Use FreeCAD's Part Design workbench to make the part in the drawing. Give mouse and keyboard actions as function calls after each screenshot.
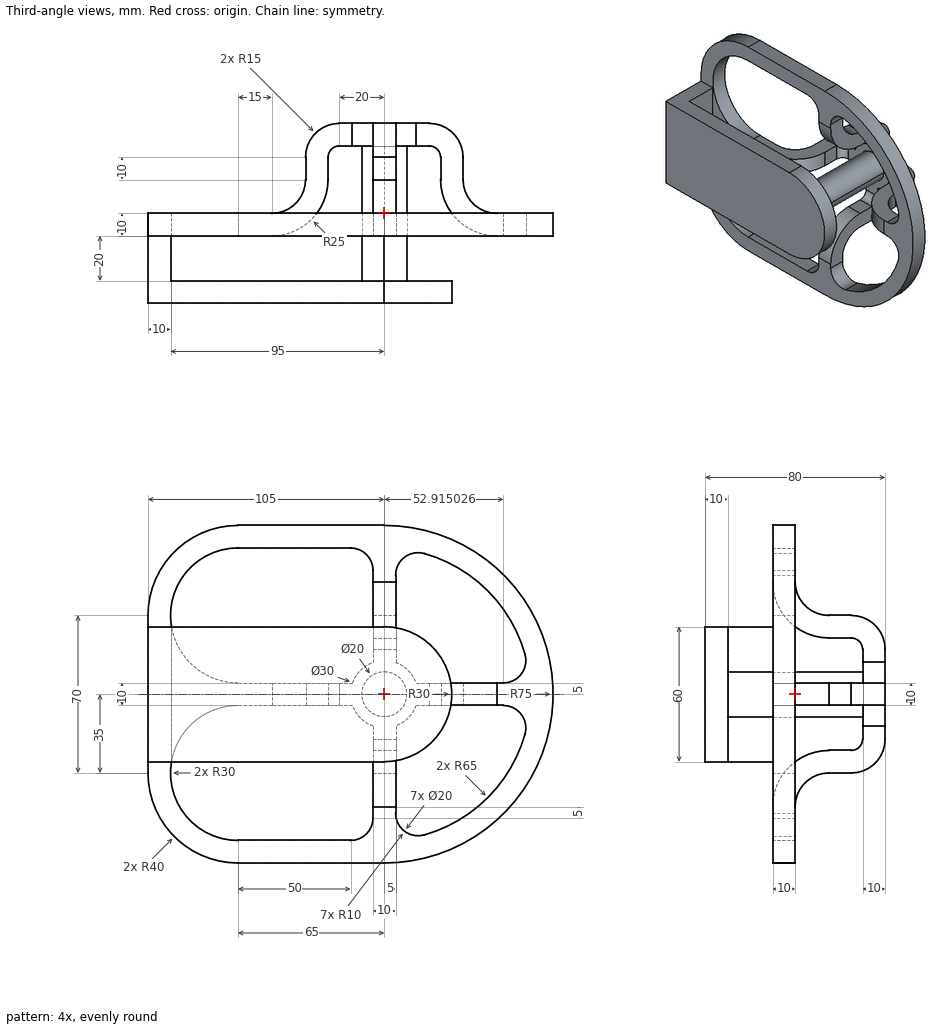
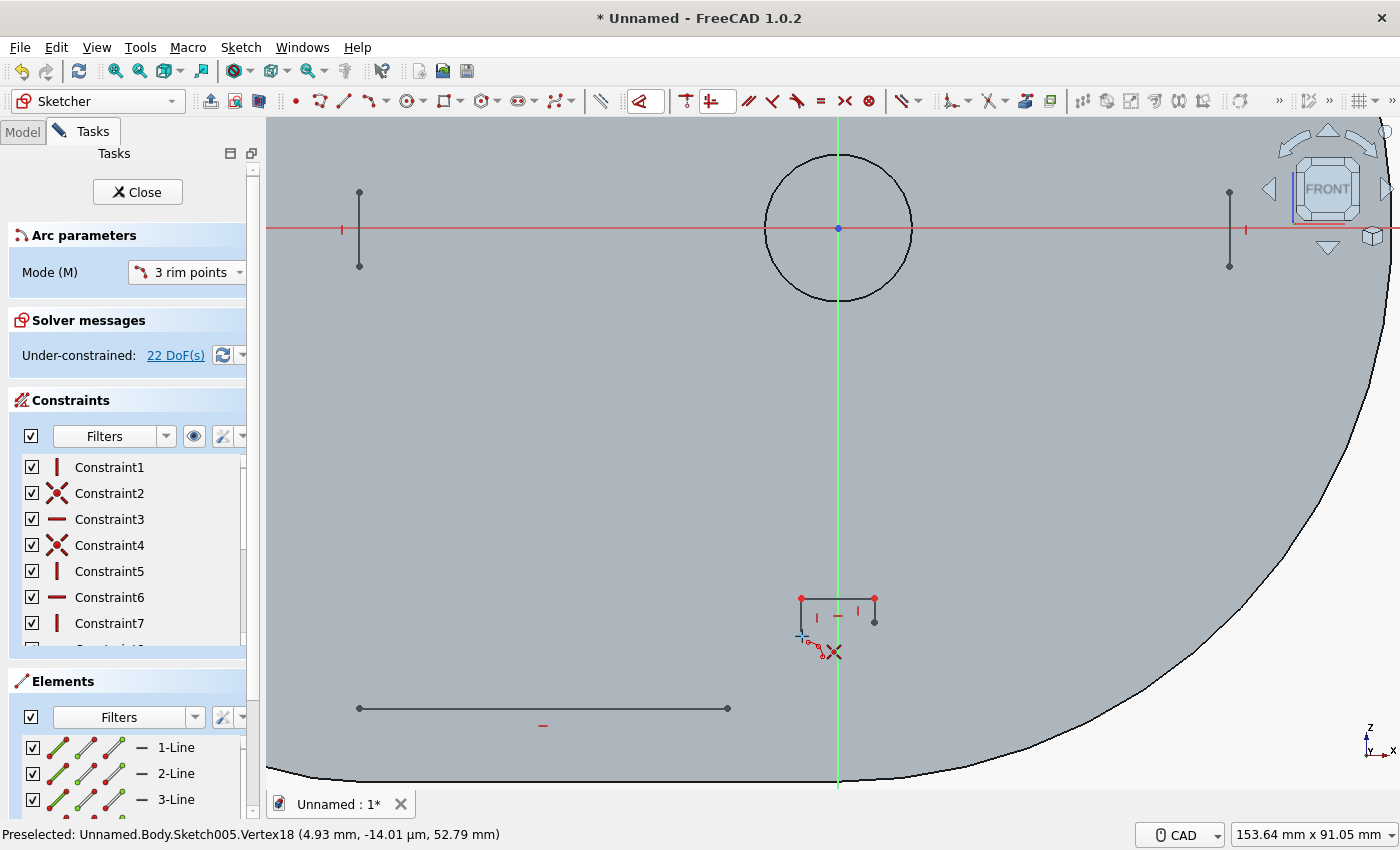
click(801, 635)
click(728, 709)
click(780, 686)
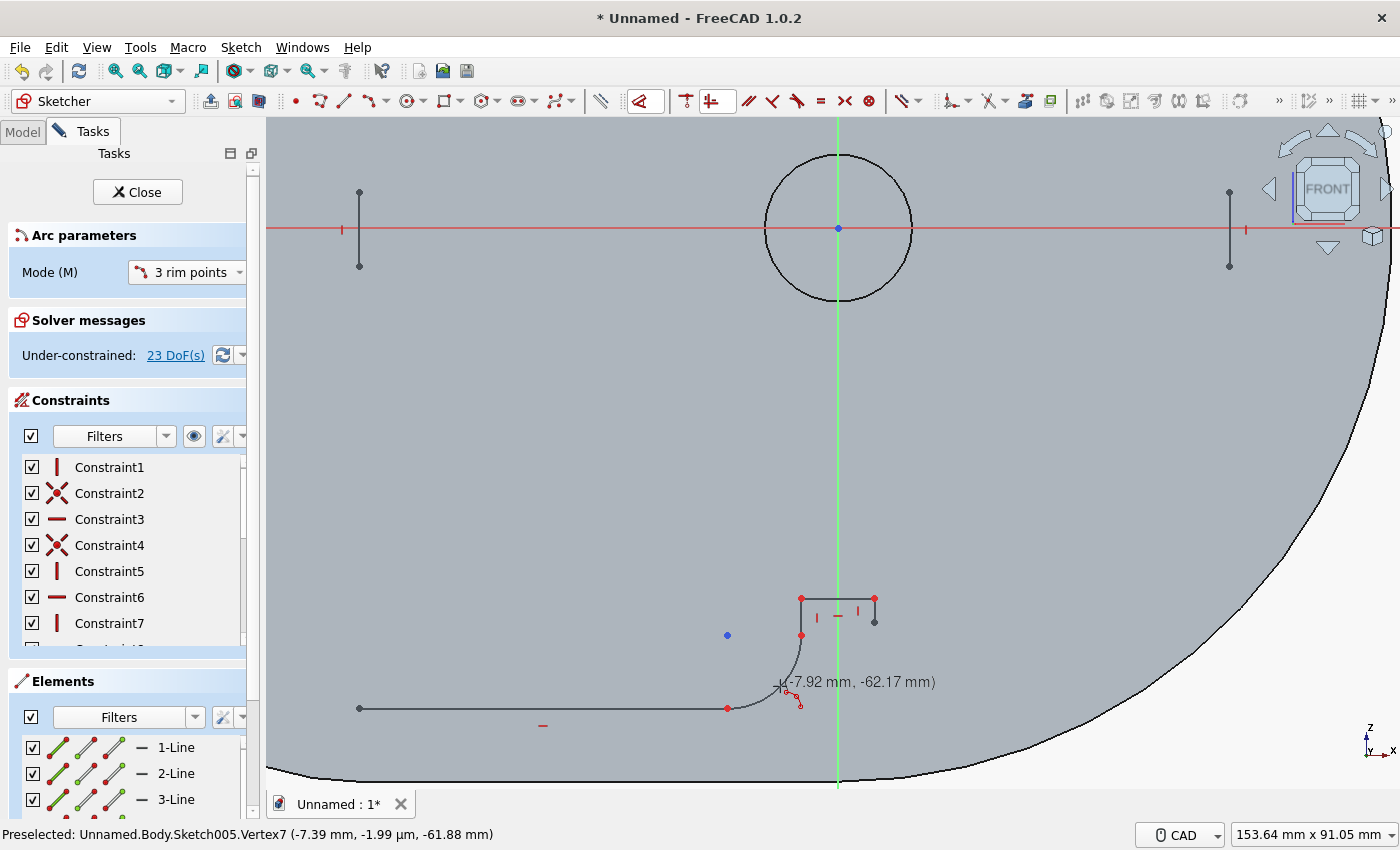
click(359, 709)
click(359, 267)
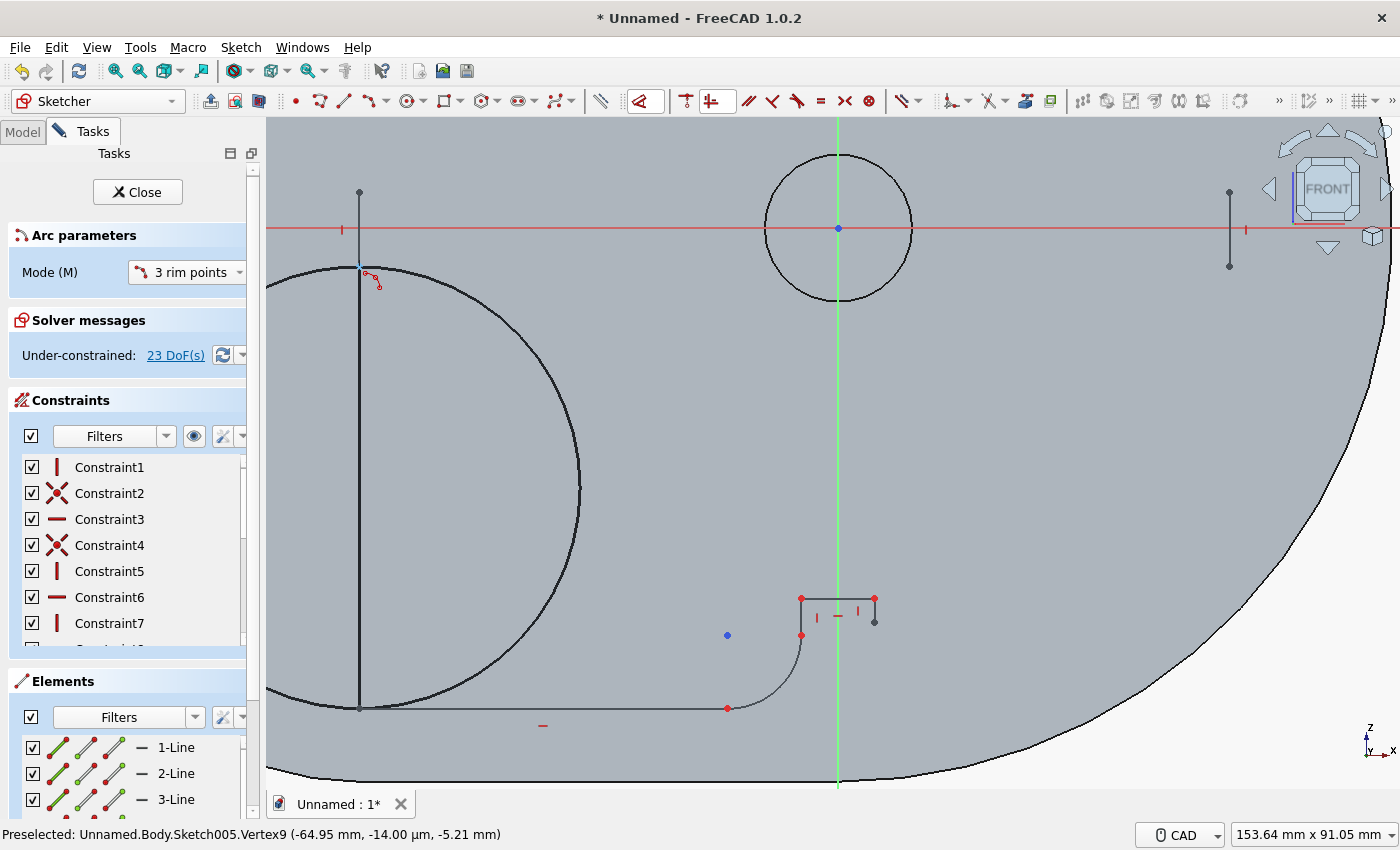
scroll(802, 636, down, 4)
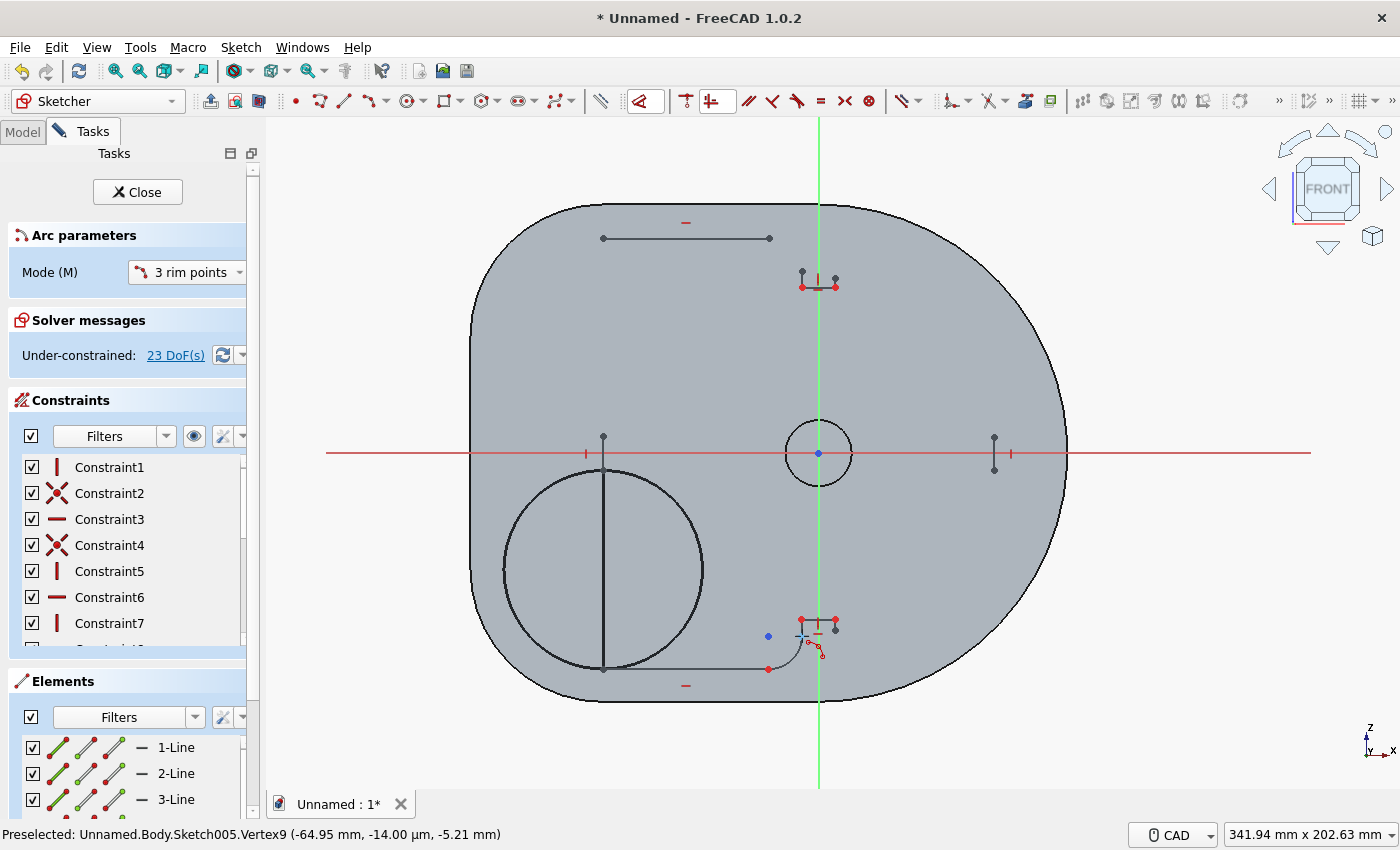
click(504, 569)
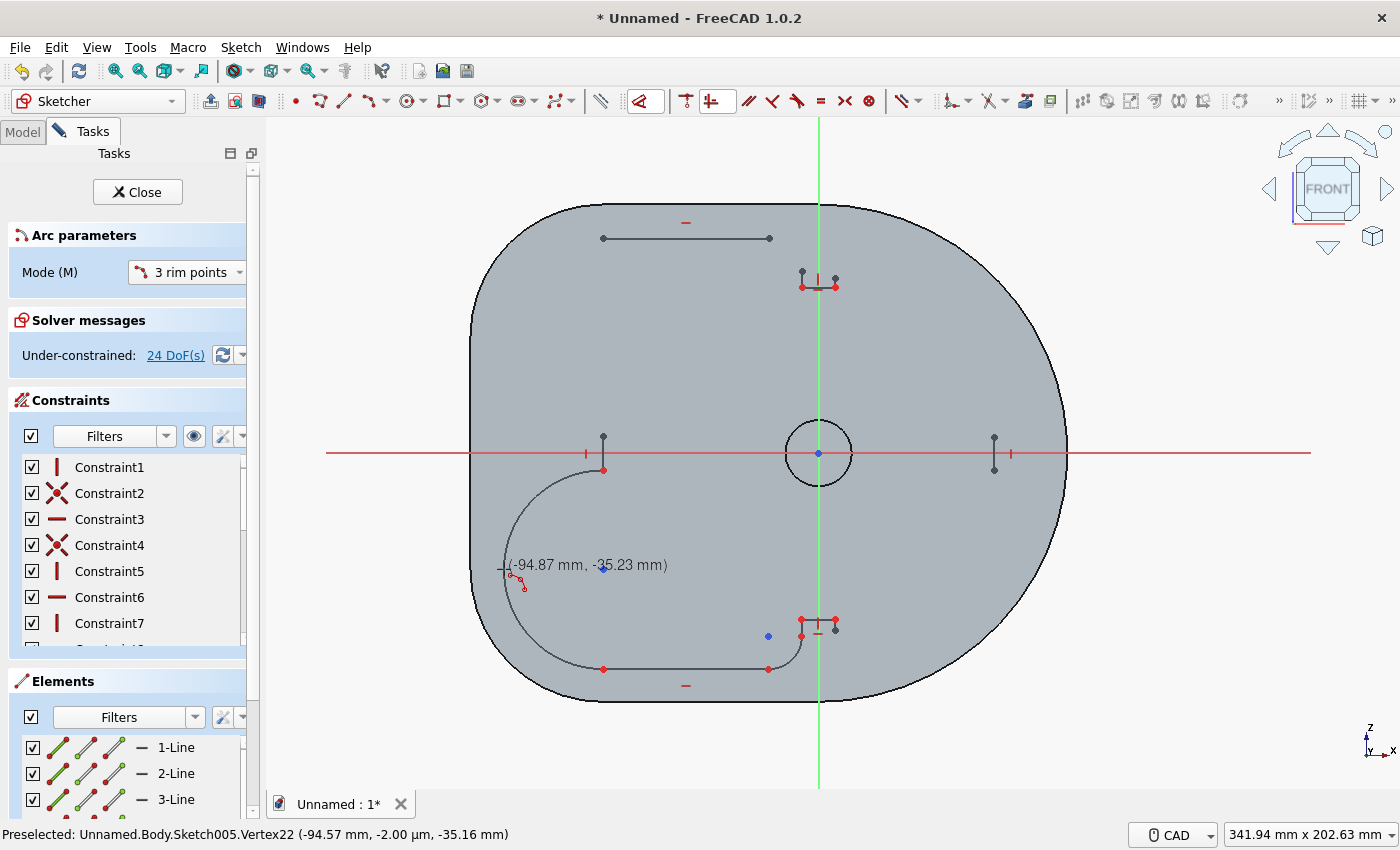
click(603, 437)
click(603, 239)
click(504, 337)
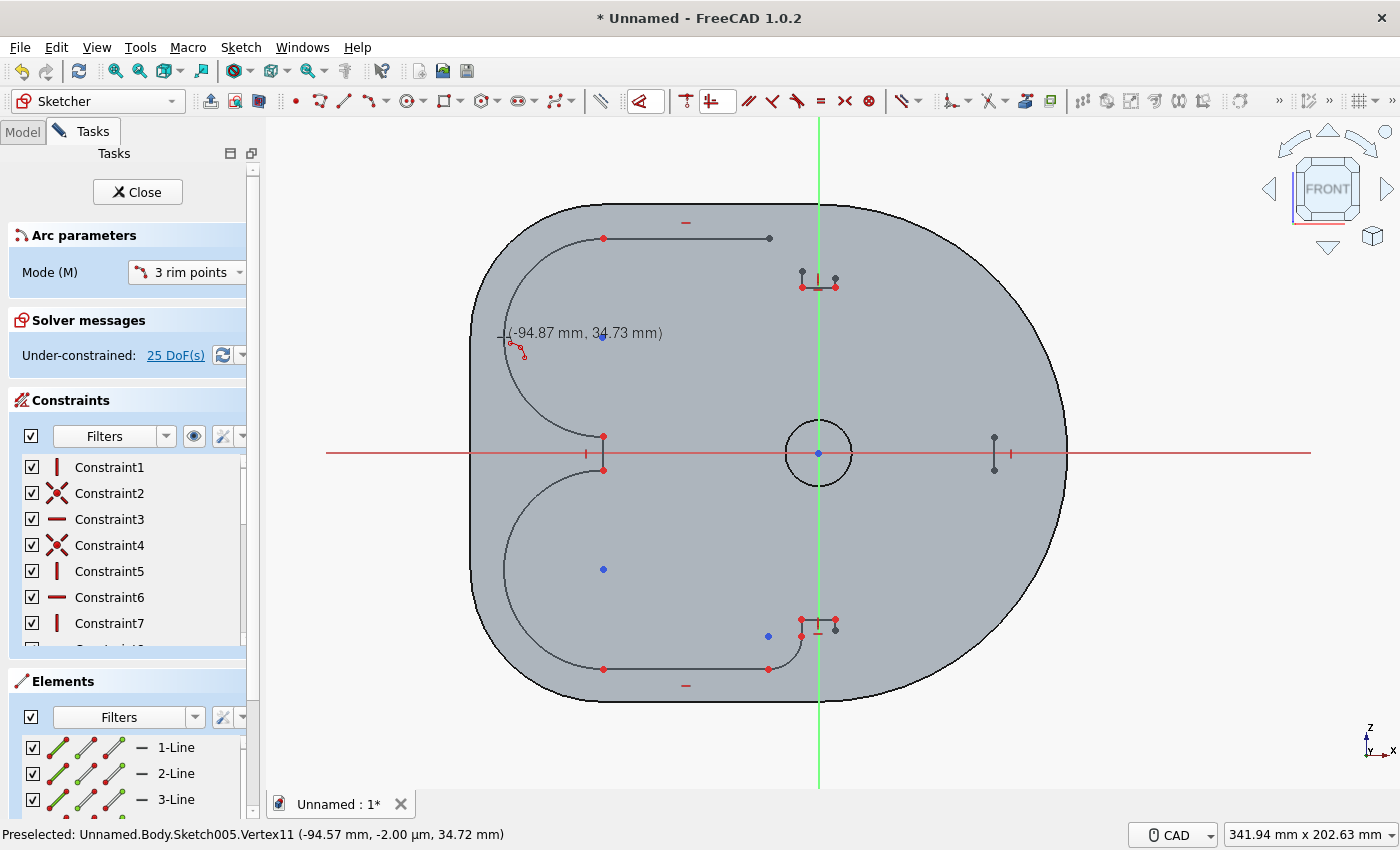
click(769, 239)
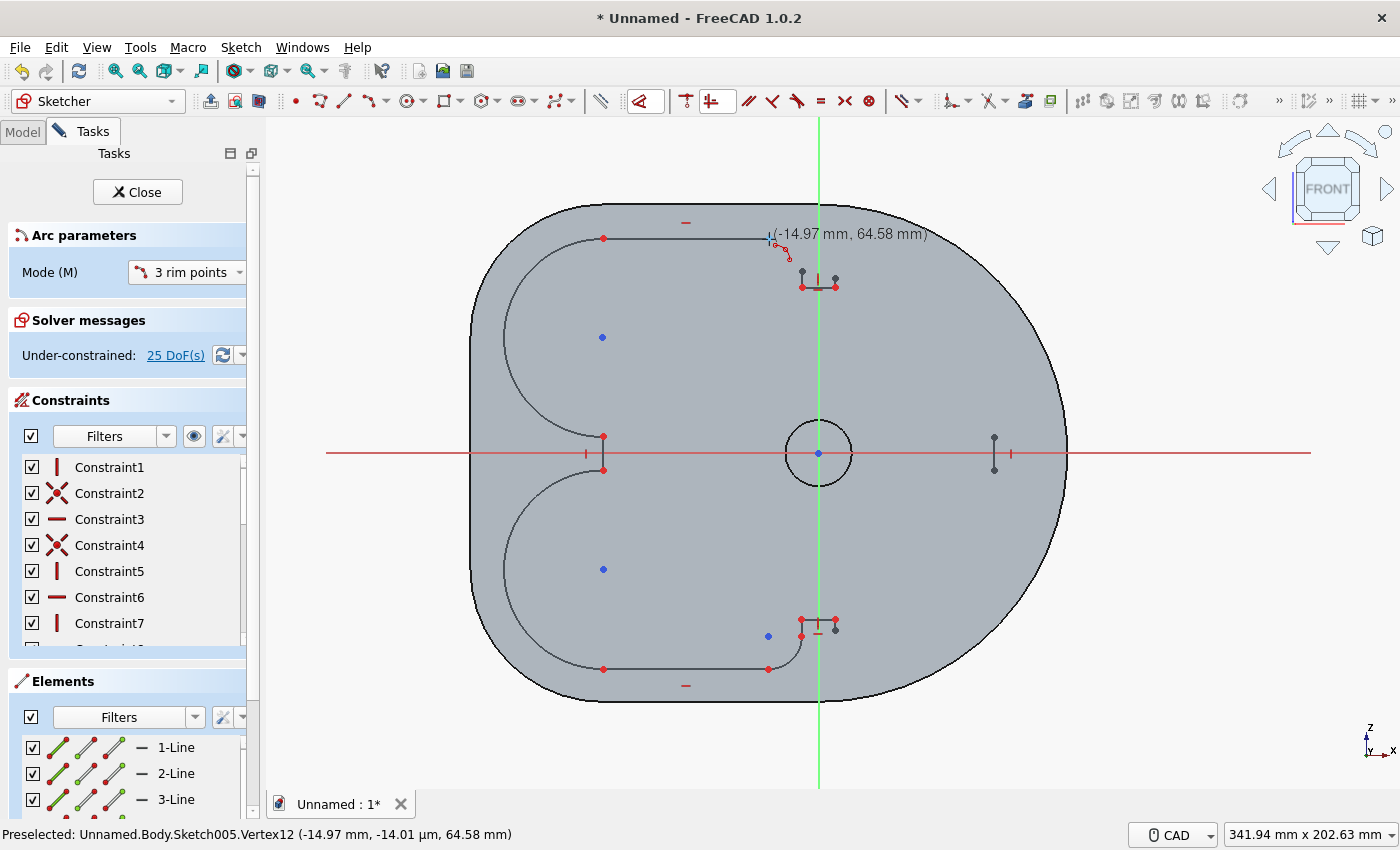
scroll(802, 271, up, 4)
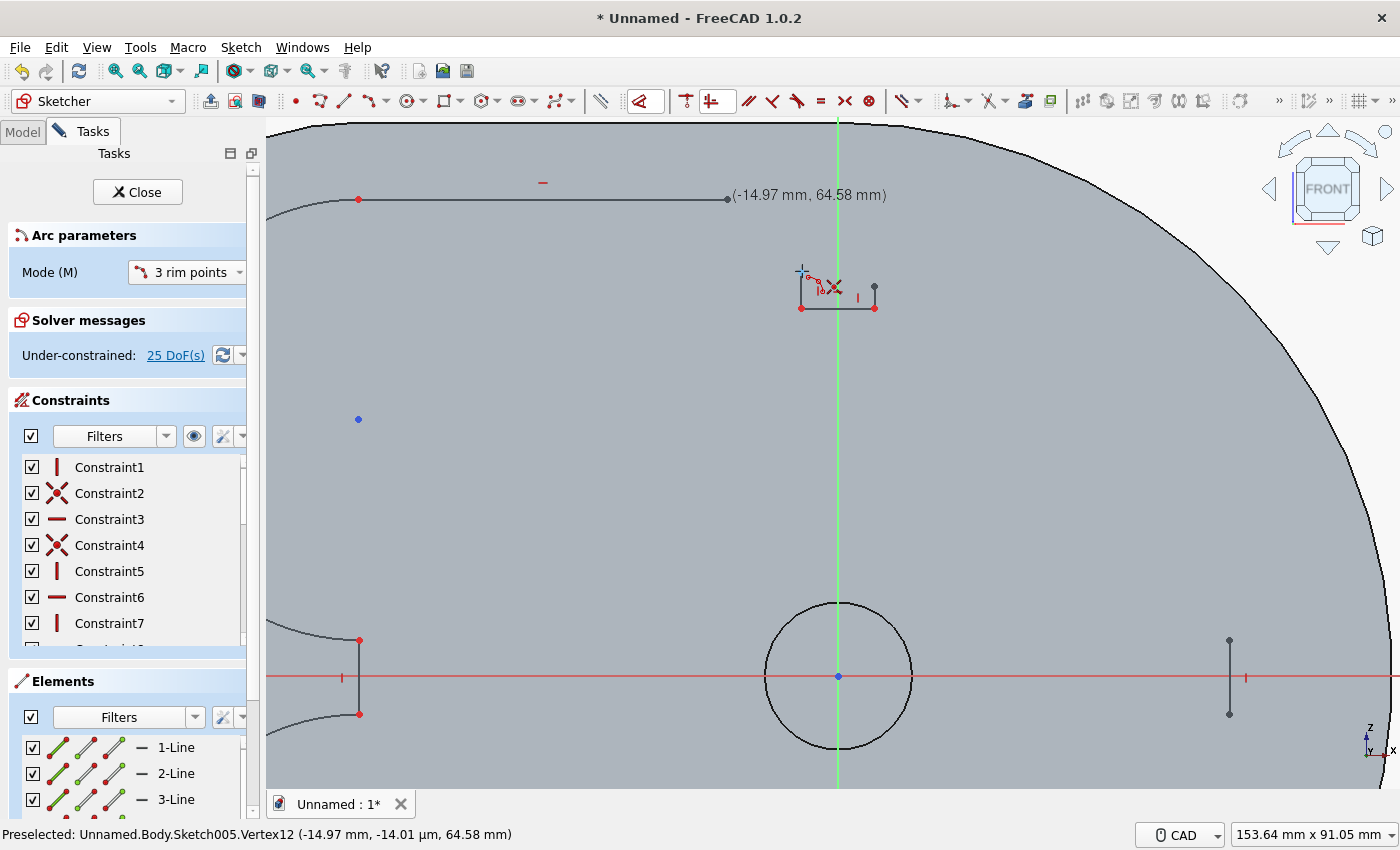
click(801, 273)
click(780, 218)